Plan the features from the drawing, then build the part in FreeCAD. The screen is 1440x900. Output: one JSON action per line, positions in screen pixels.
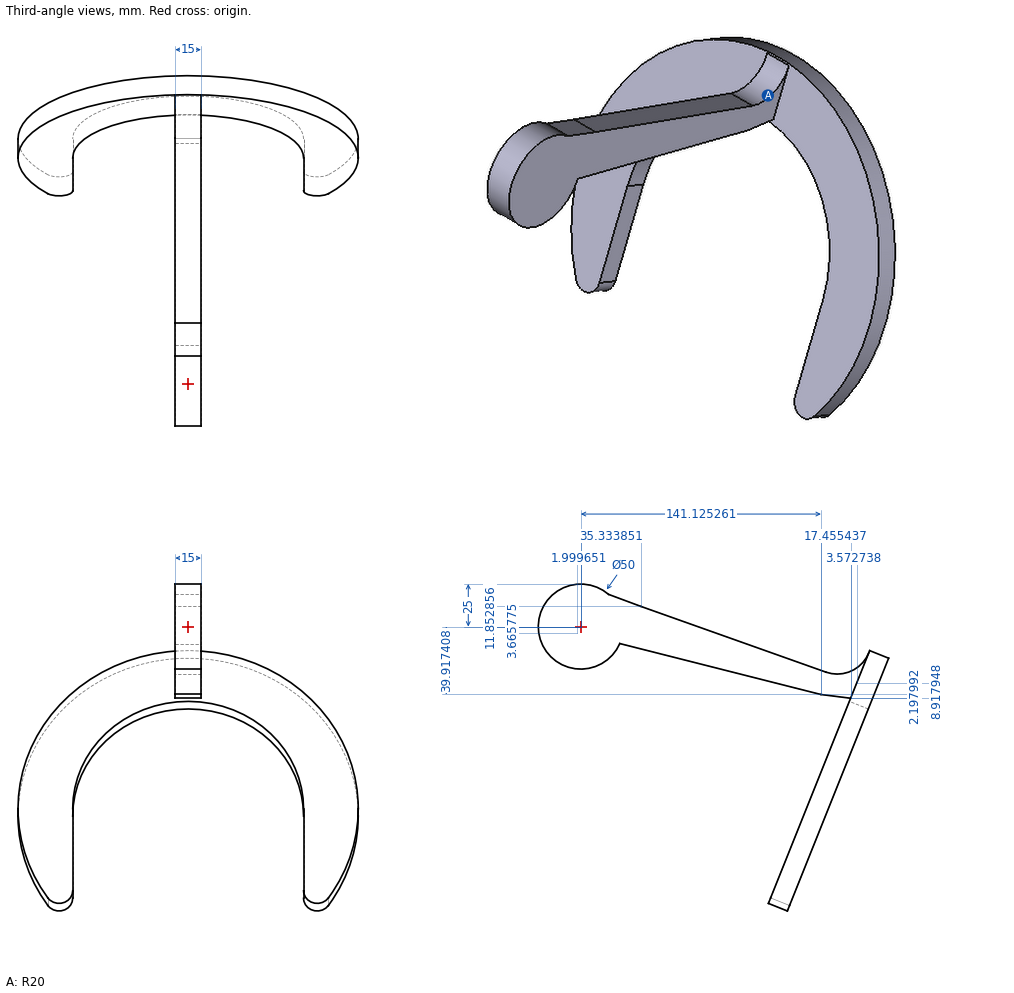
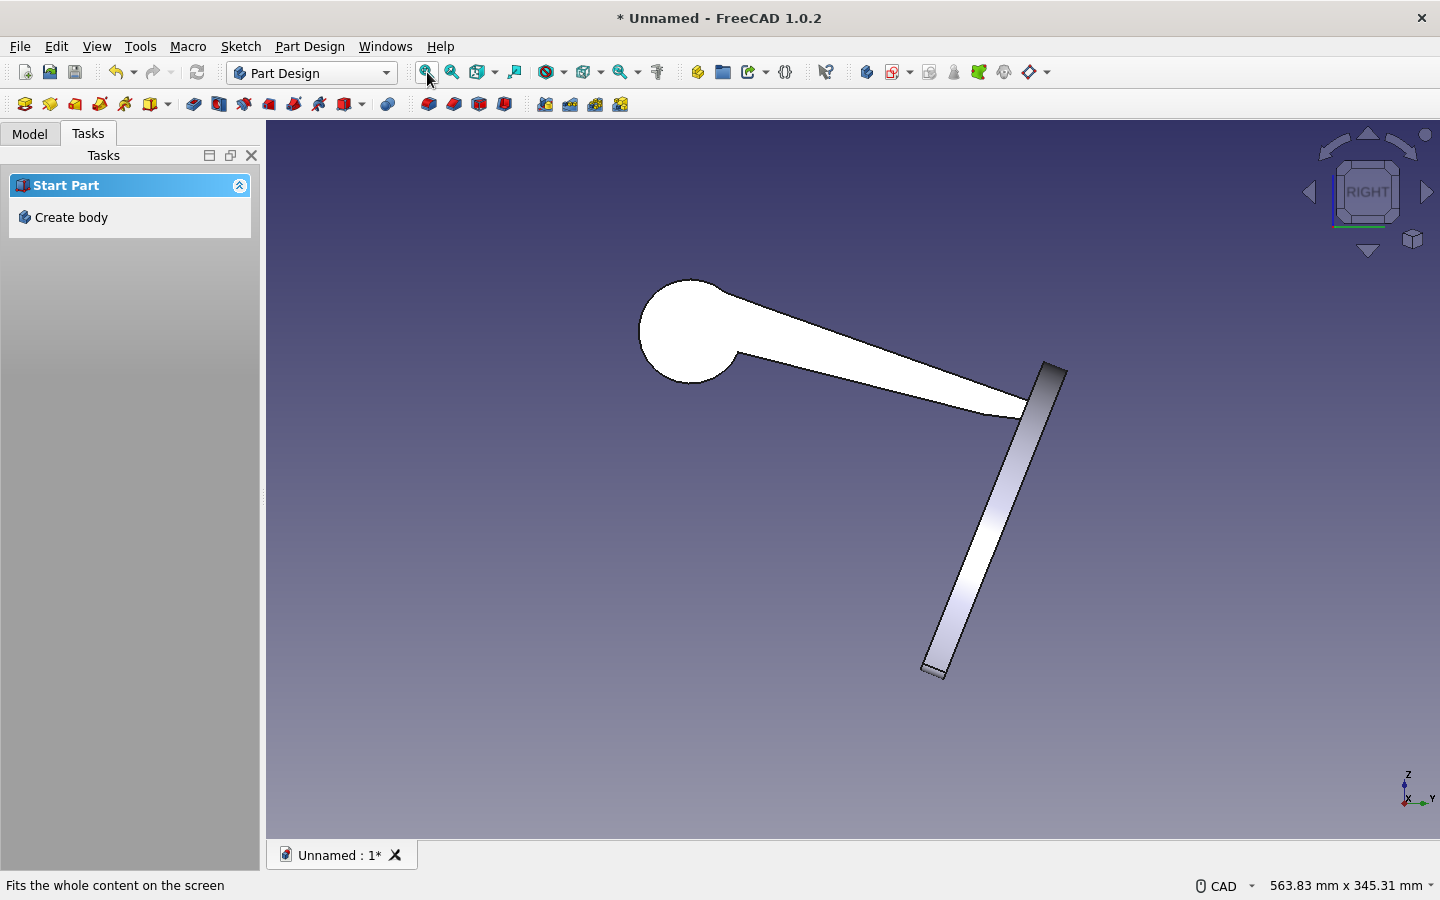
{"action": "key", "text": "5"}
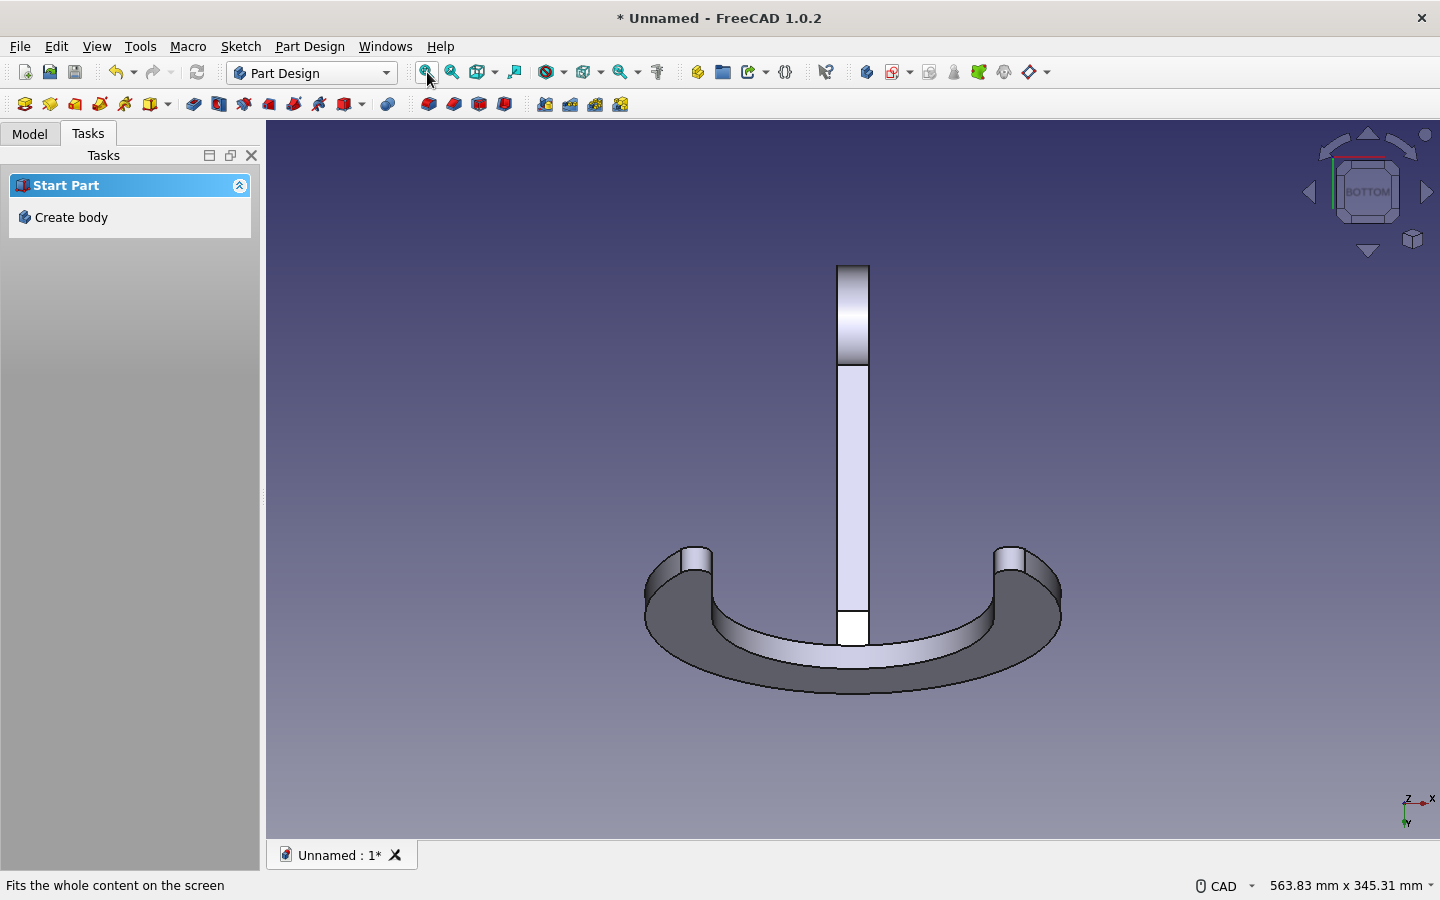
{"action": "key", "text": "4"}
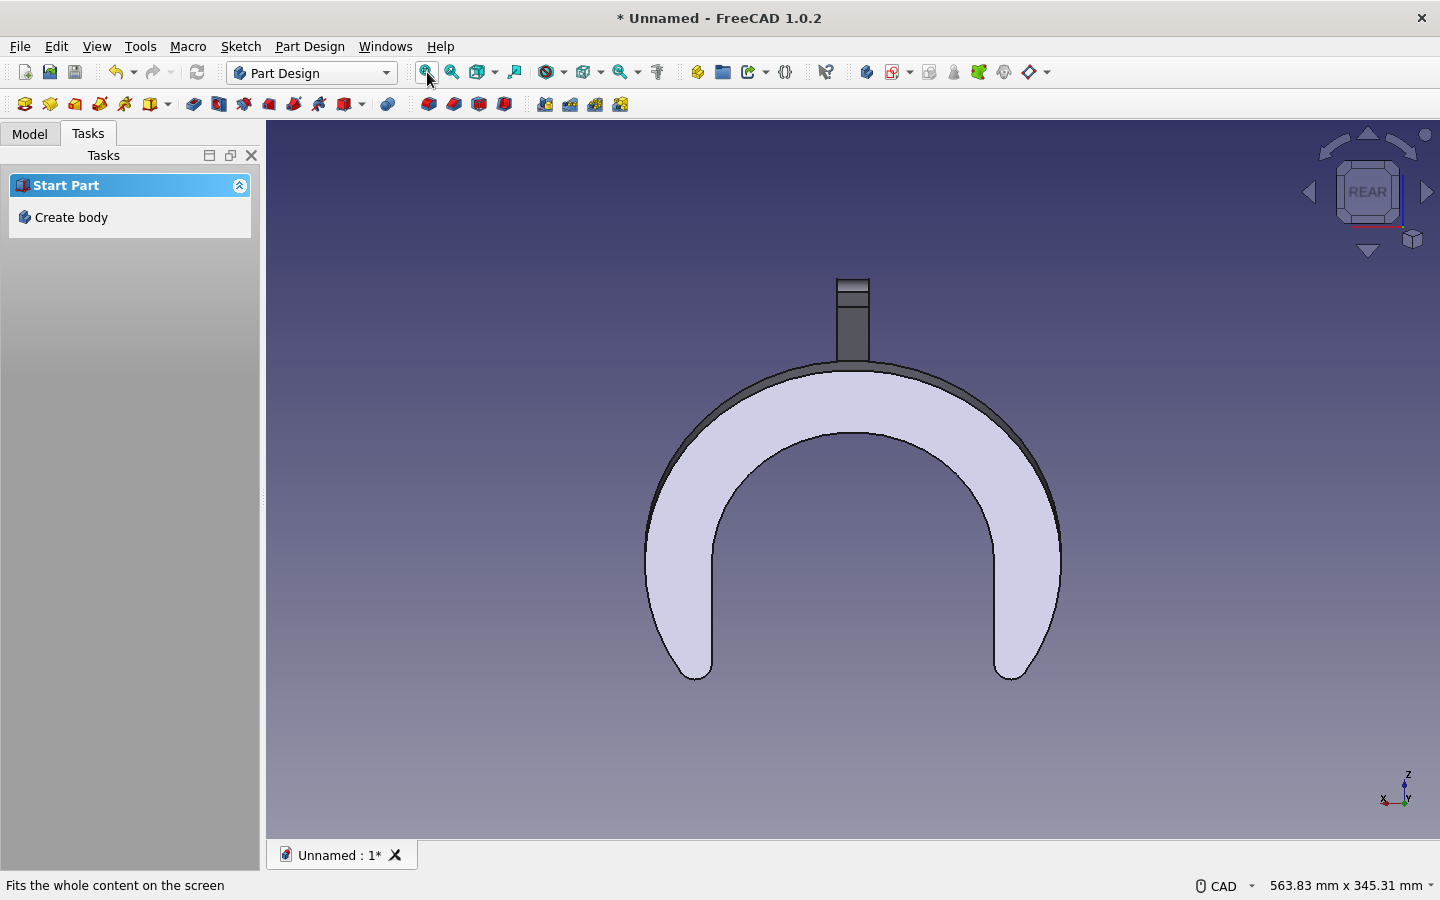
{"action": "key", "text": "6"}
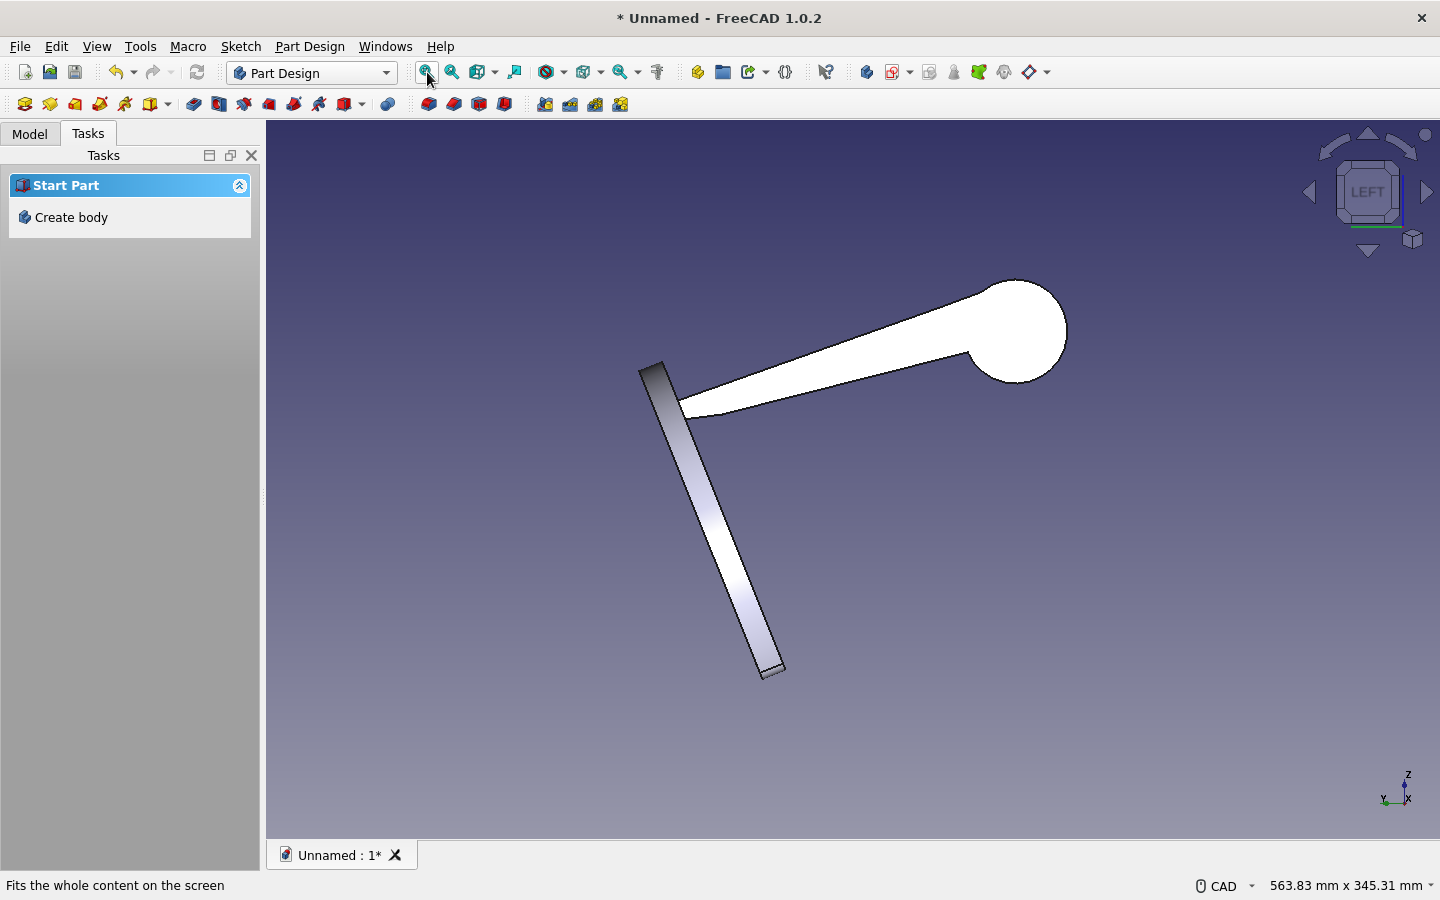
{"action": "key", "text": "v 3"}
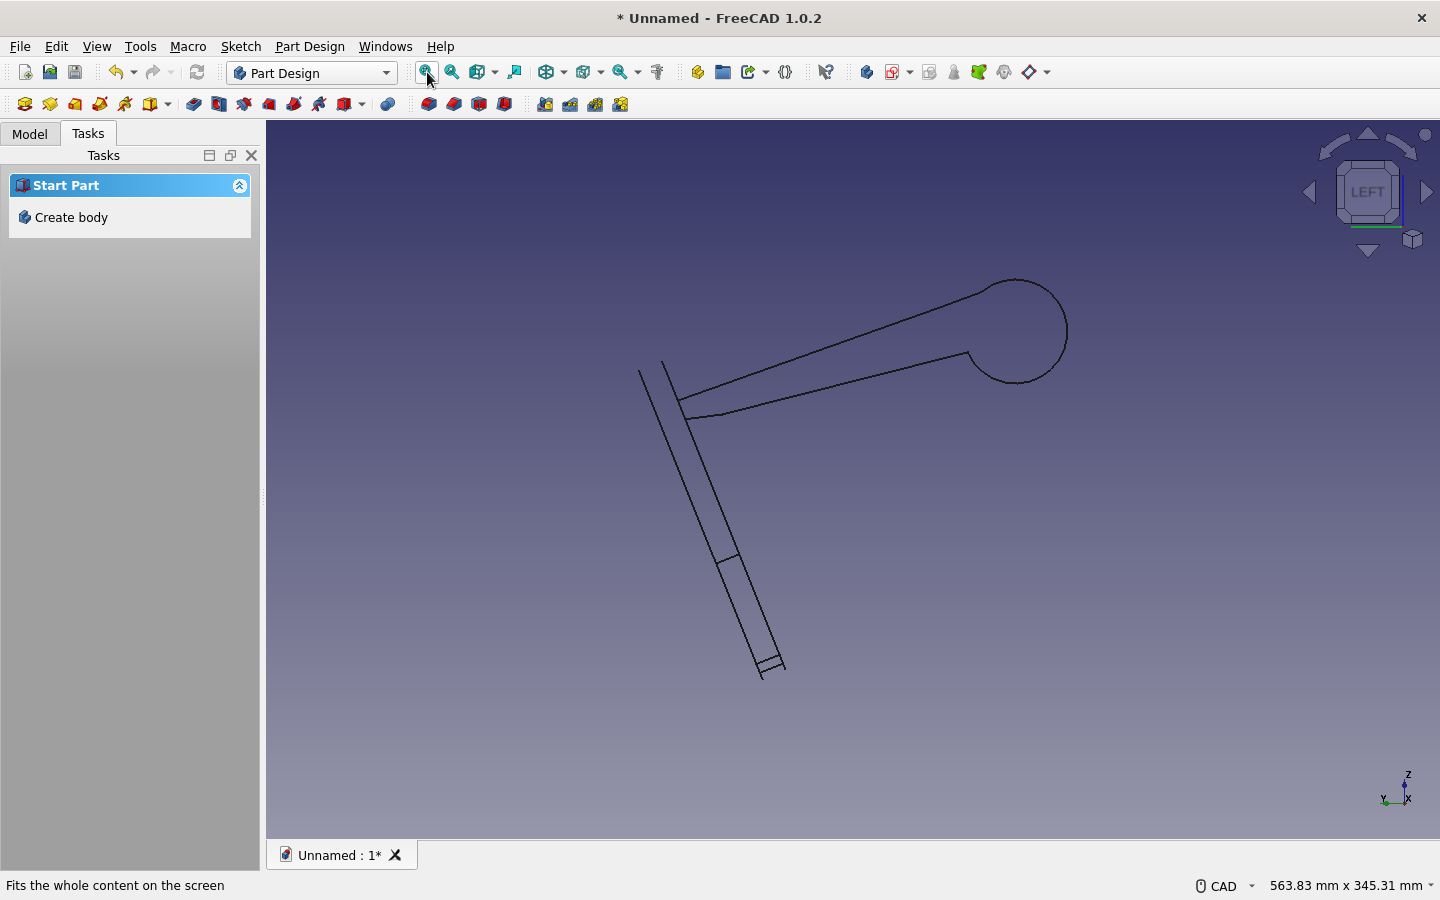
{"action": "key", "text": "0"}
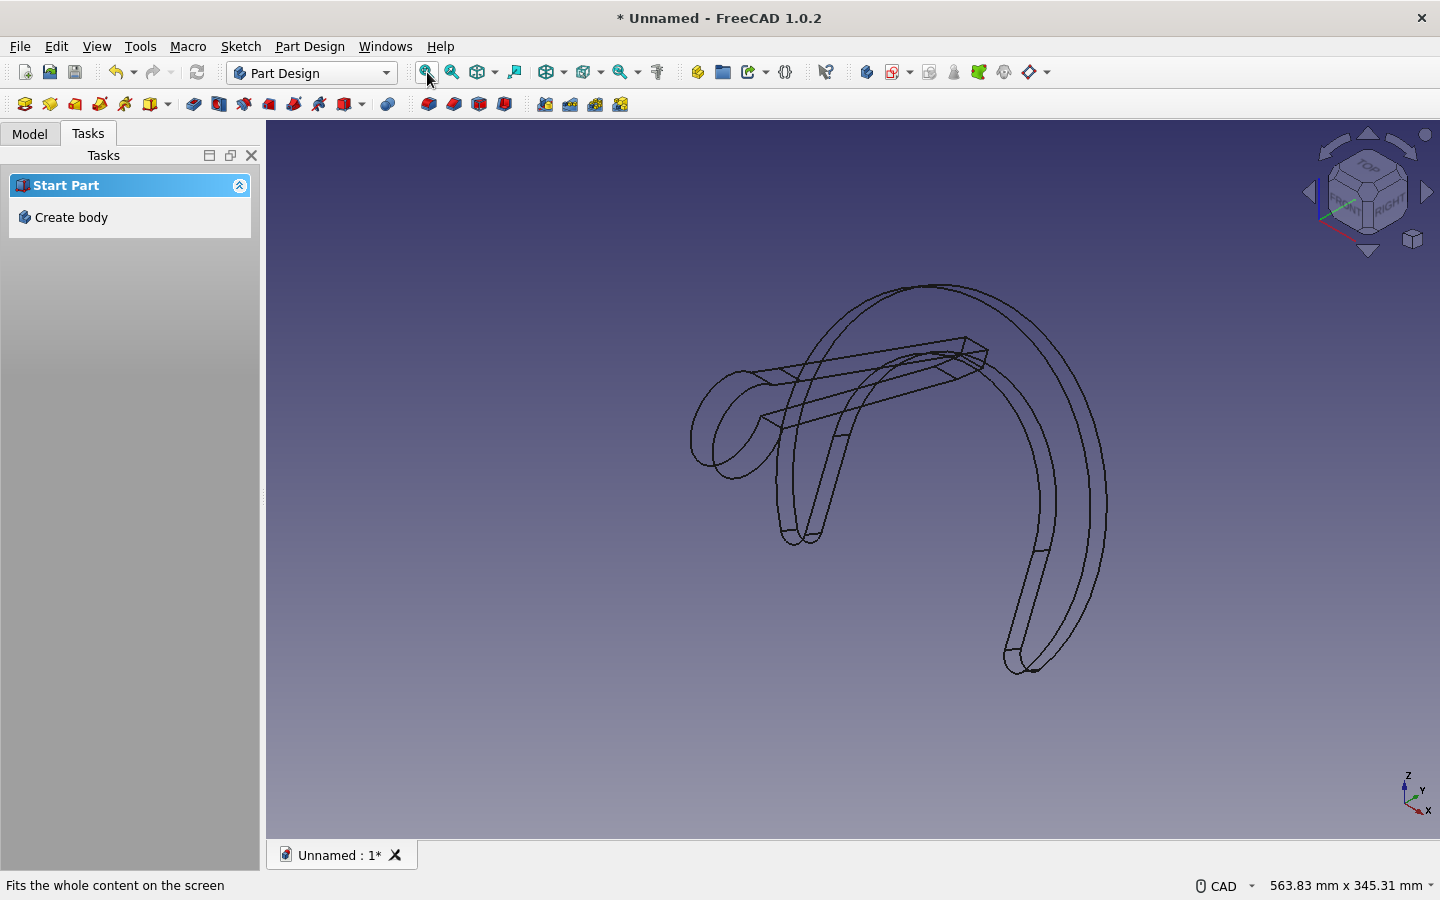
{"action": "left_click", "coordinate": [977, 343]}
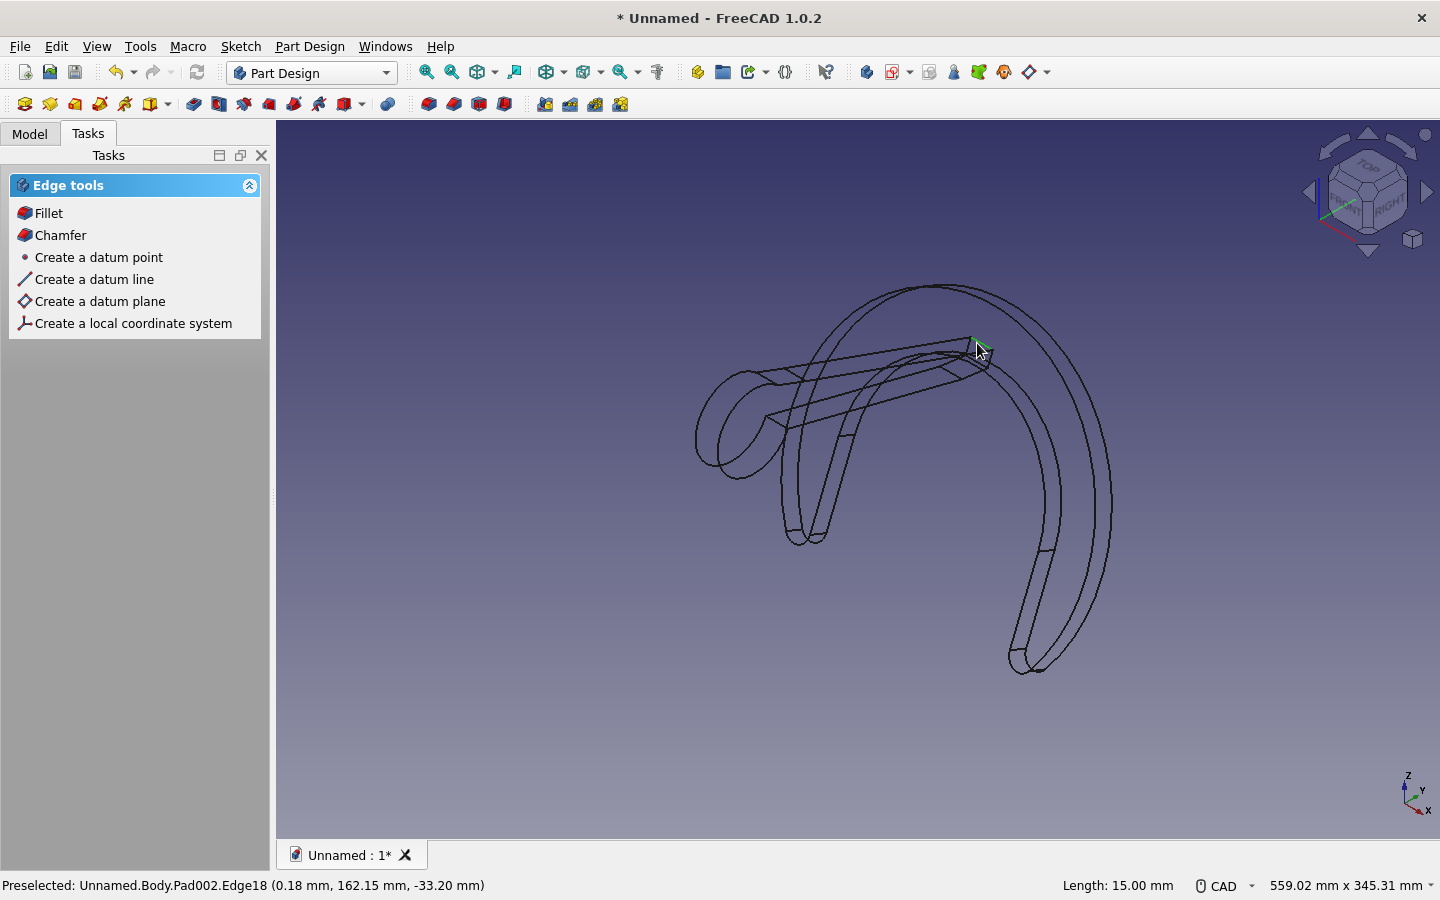
{"action": "key", "text": "v 1"}